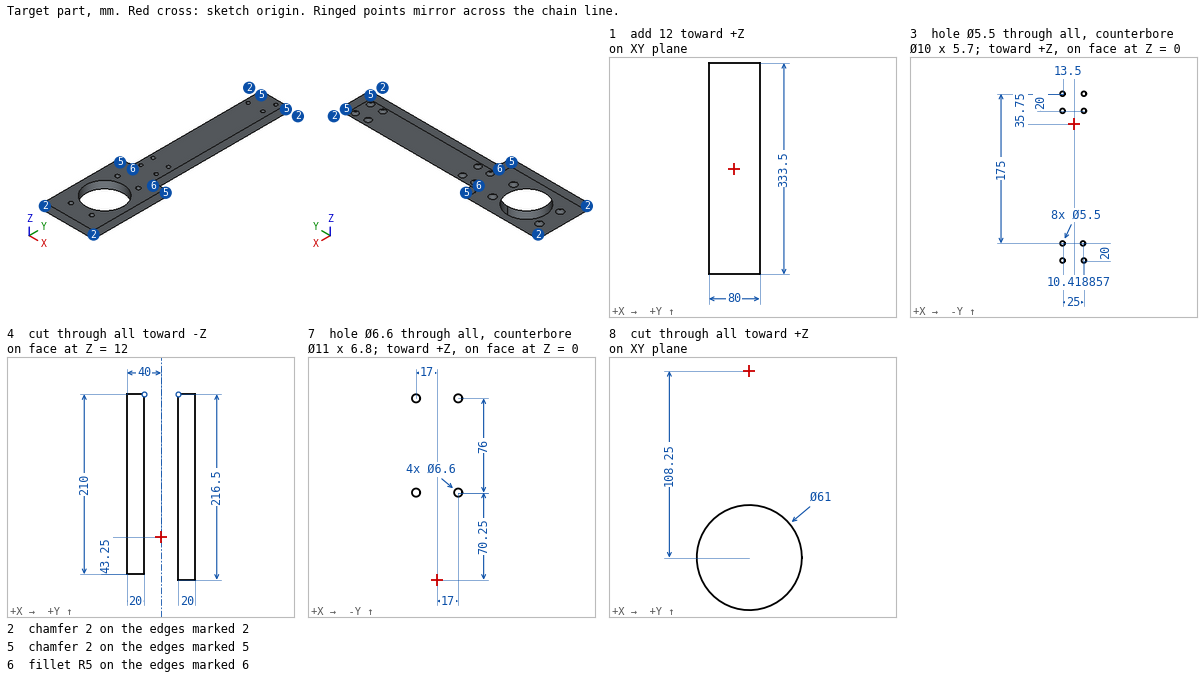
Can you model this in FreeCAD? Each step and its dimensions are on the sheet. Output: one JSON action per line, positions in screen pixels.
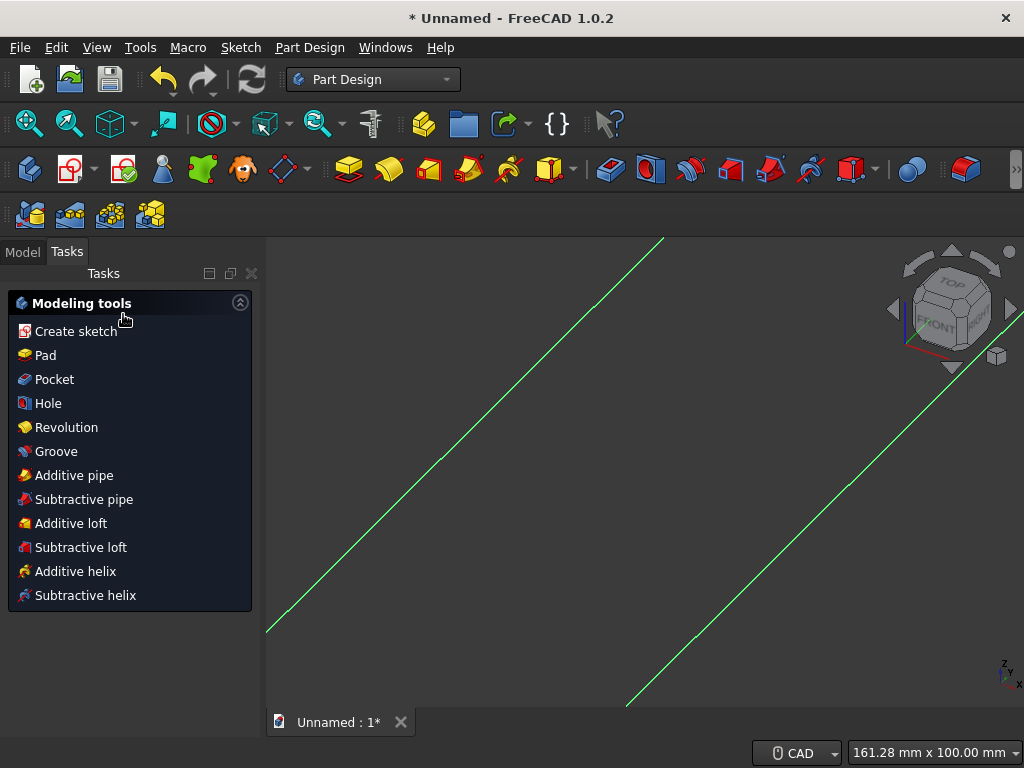
{"action": "left_click", "coordinate": [350, 170]}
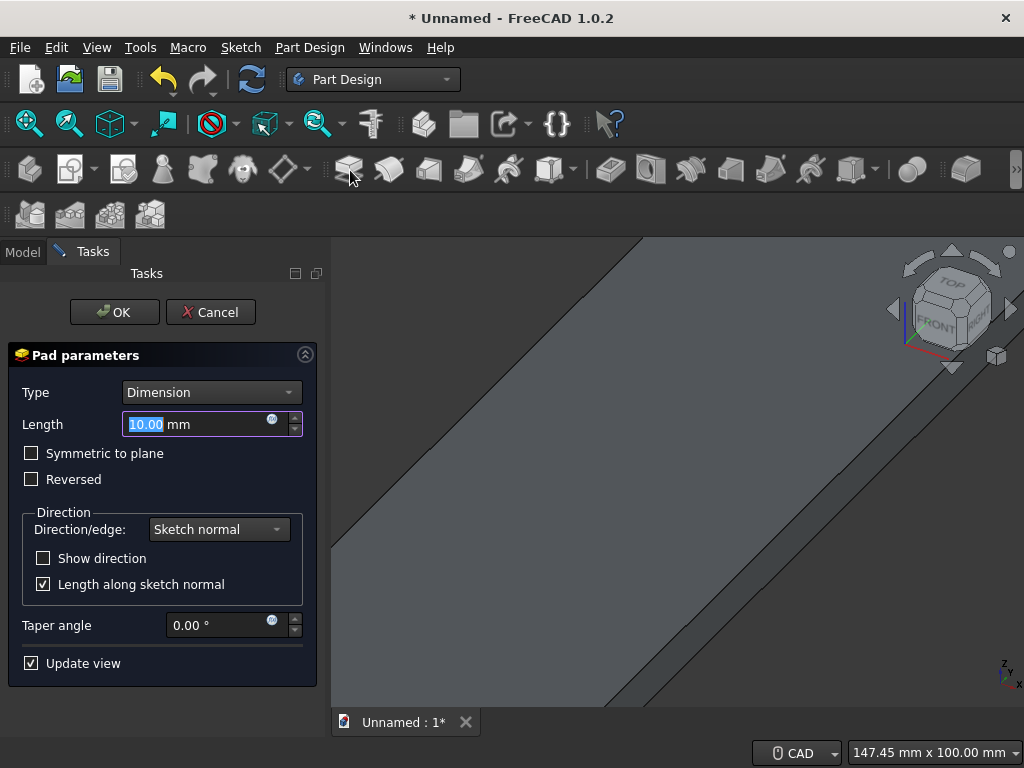
{"action": "type", "text": "12"}
{"action": "key", "text": "Tab"}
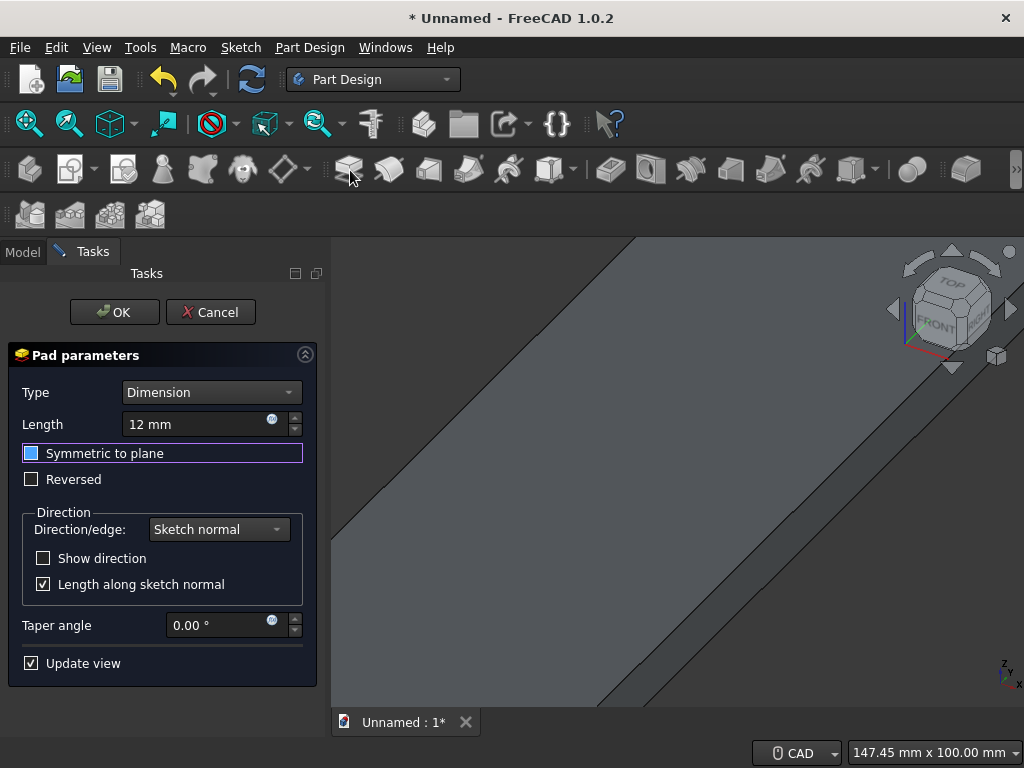
{"action": "left_click", "coordinate": [115, 312]}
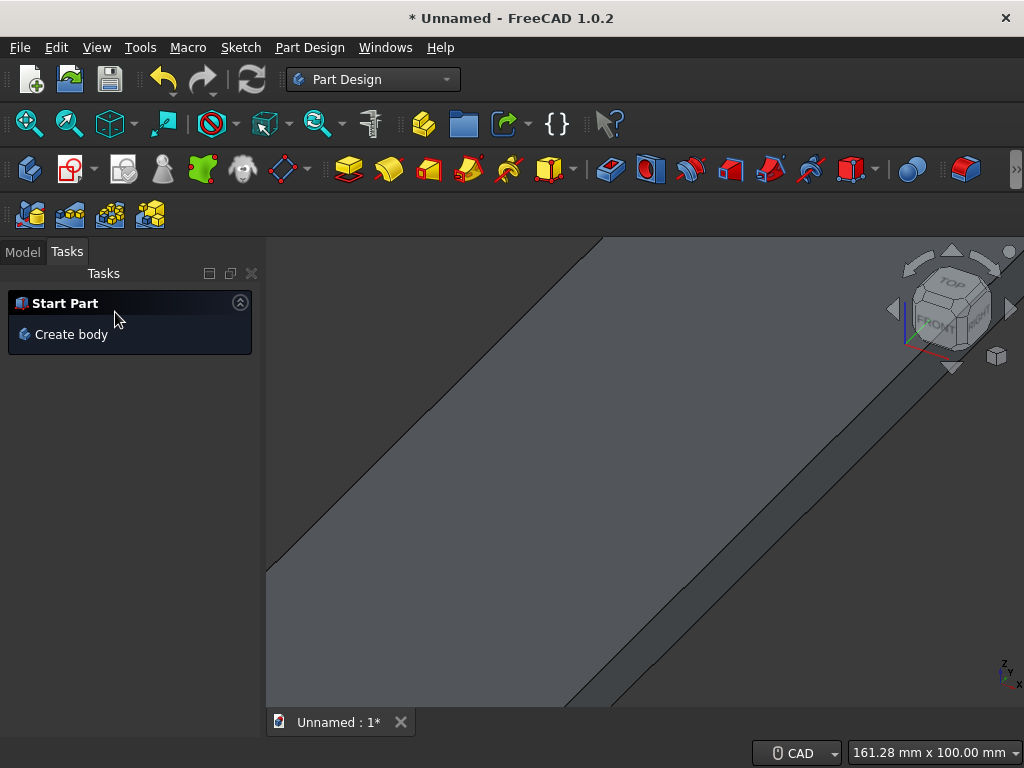
{"action": "left_click", "coordinate": [30, 124]}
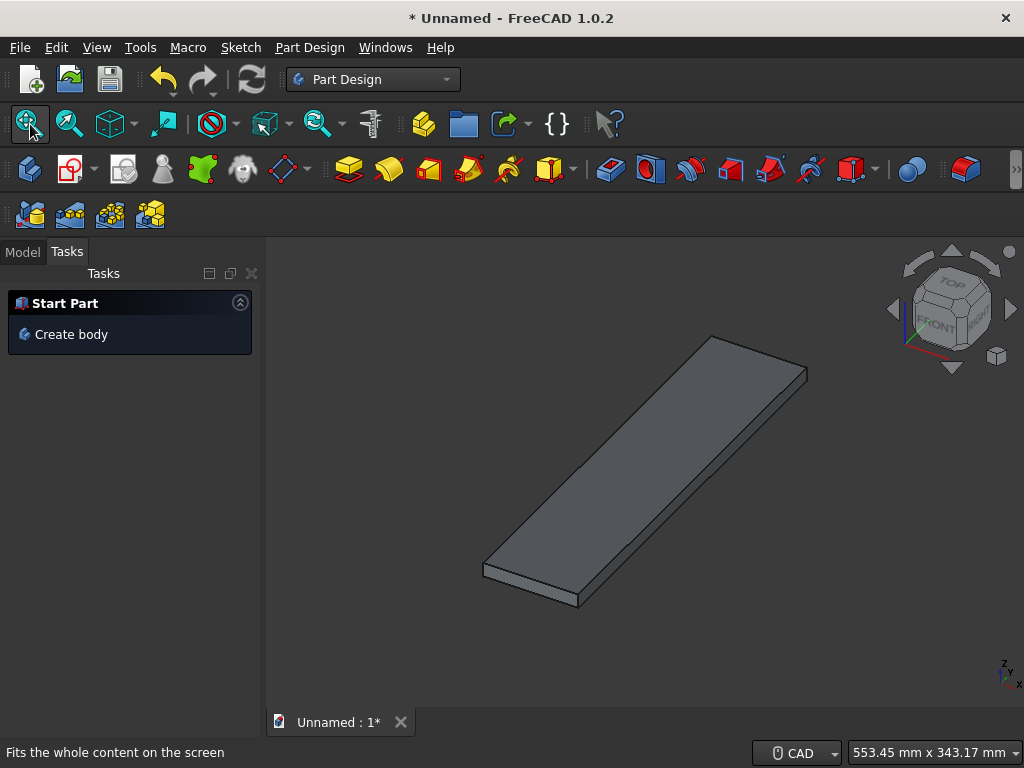
{"action": "left_click", "coordinate": [578, 600]}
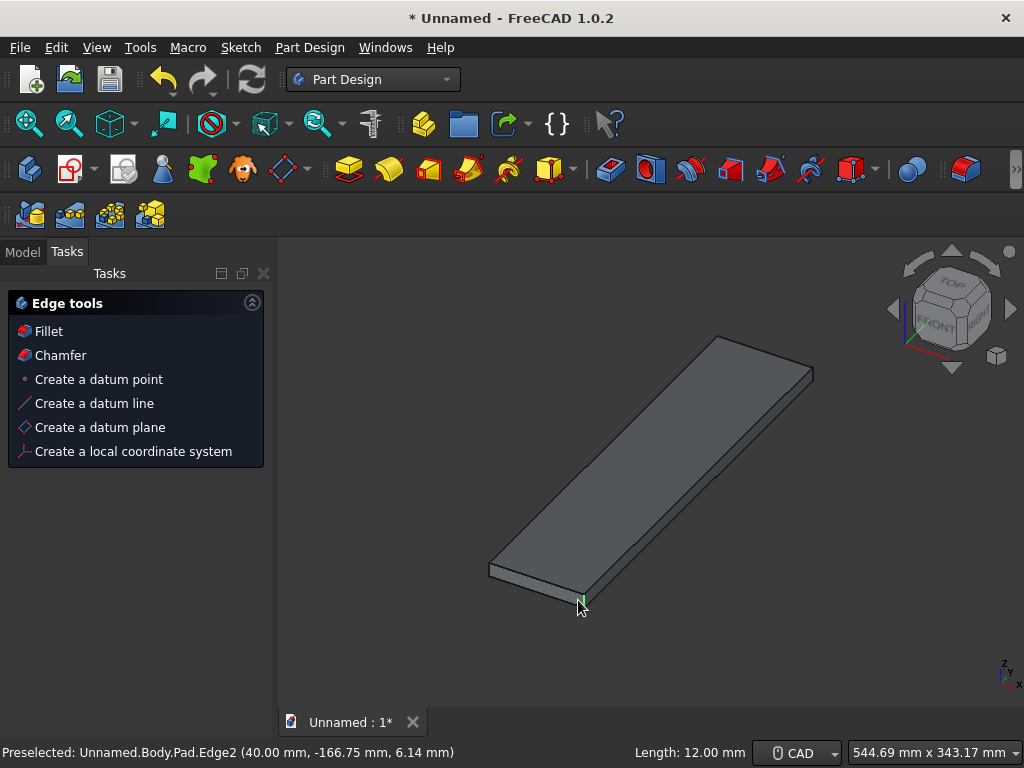
{"action": "scroll", "coordinate": [489, 569], "scroll_direction": "up", "scroll_amount": 5}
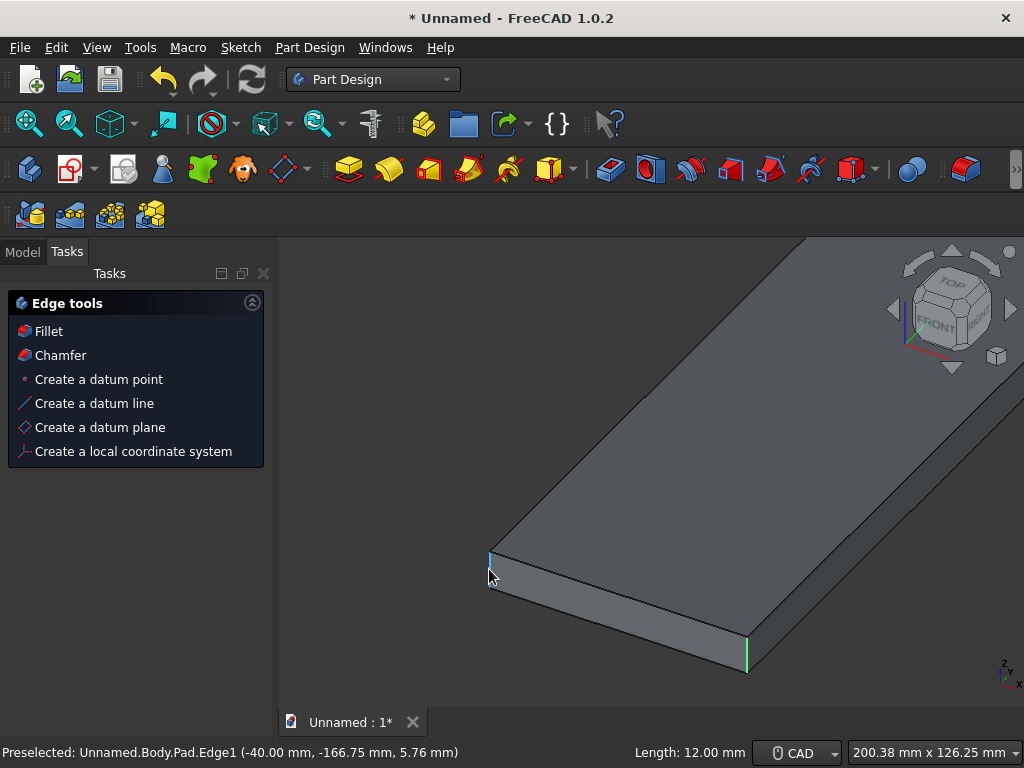
{"action": "key", "text": "v f"}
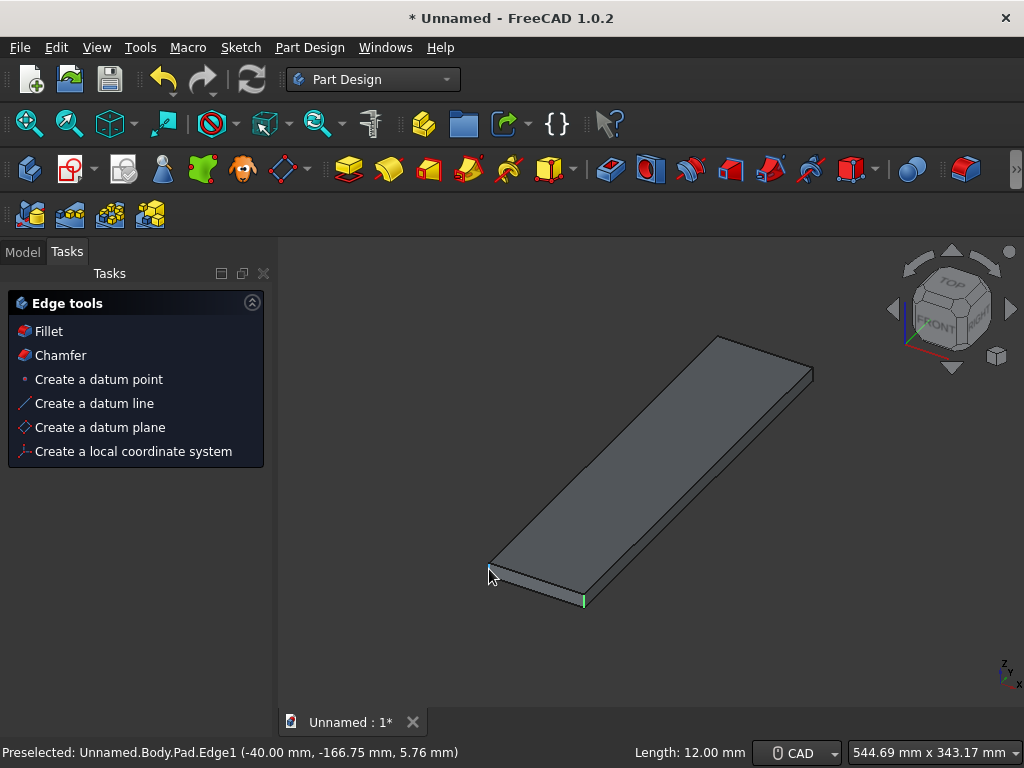
{"action": "key", "text": "0"}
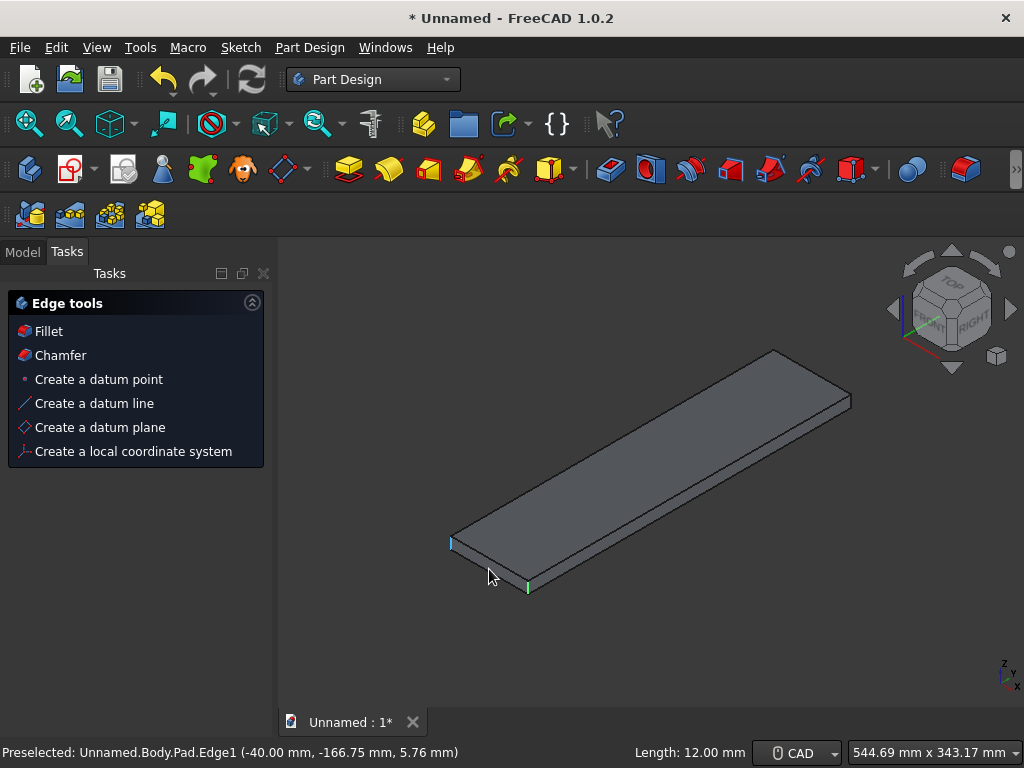
{"action": "scroll", "coordinate": [451, 542], "scroll_direction": "up", "scroll_amount": 5}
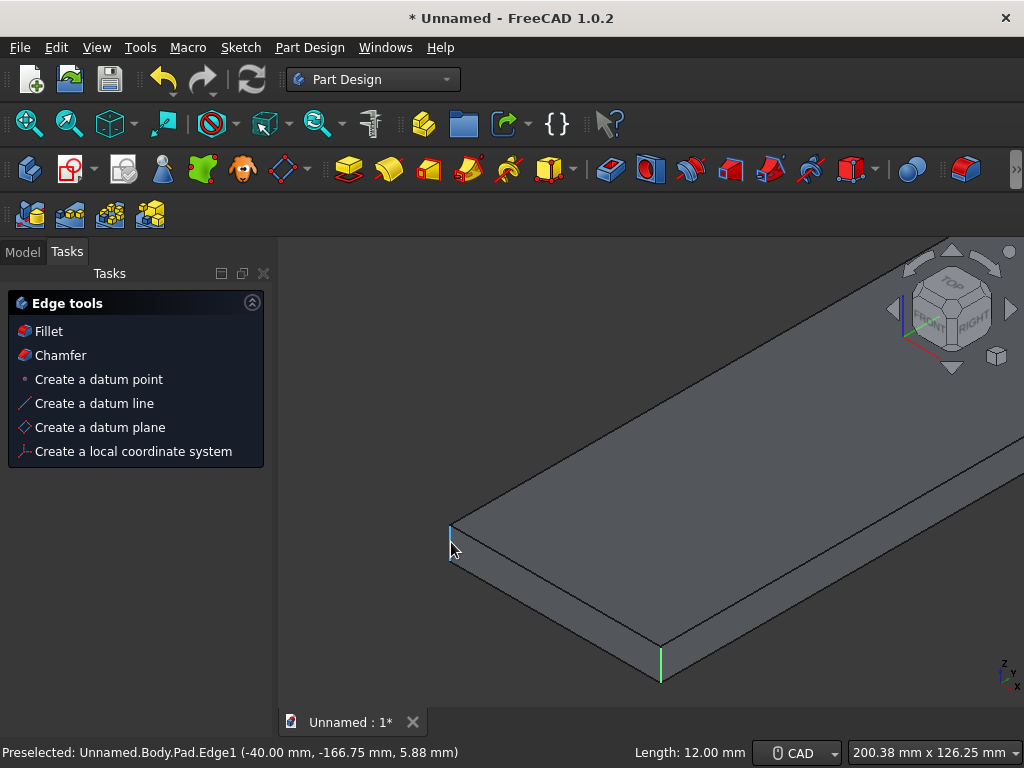
{"action": "key", "text": "v f"}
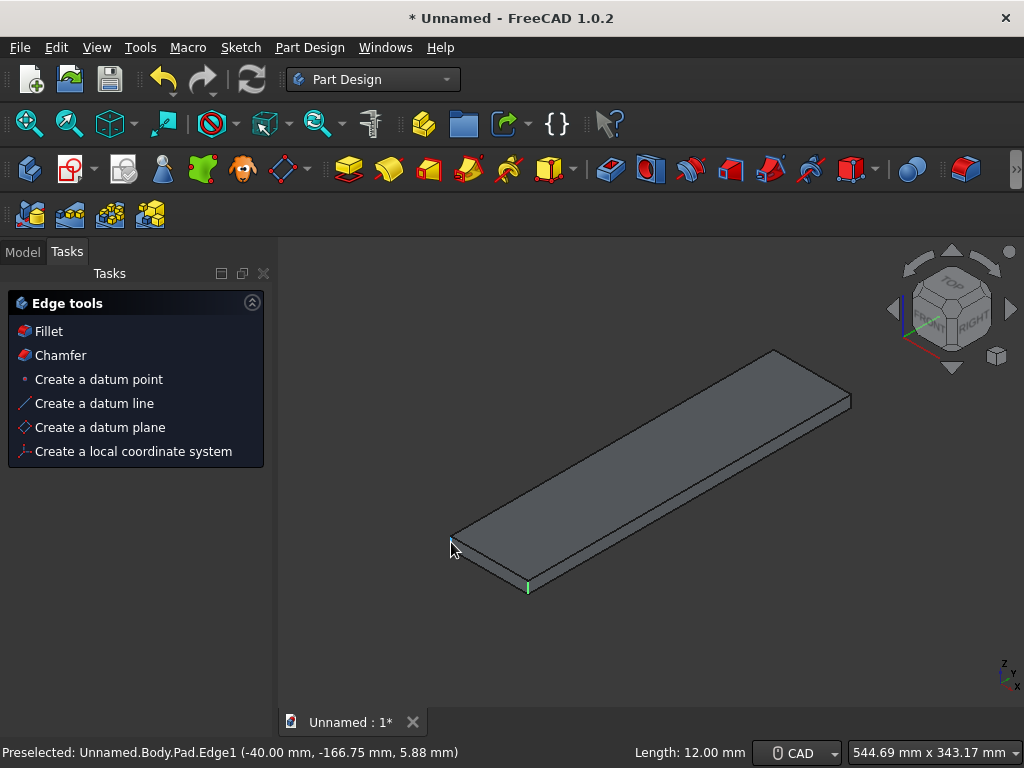
{"action": "key", "text": "2"}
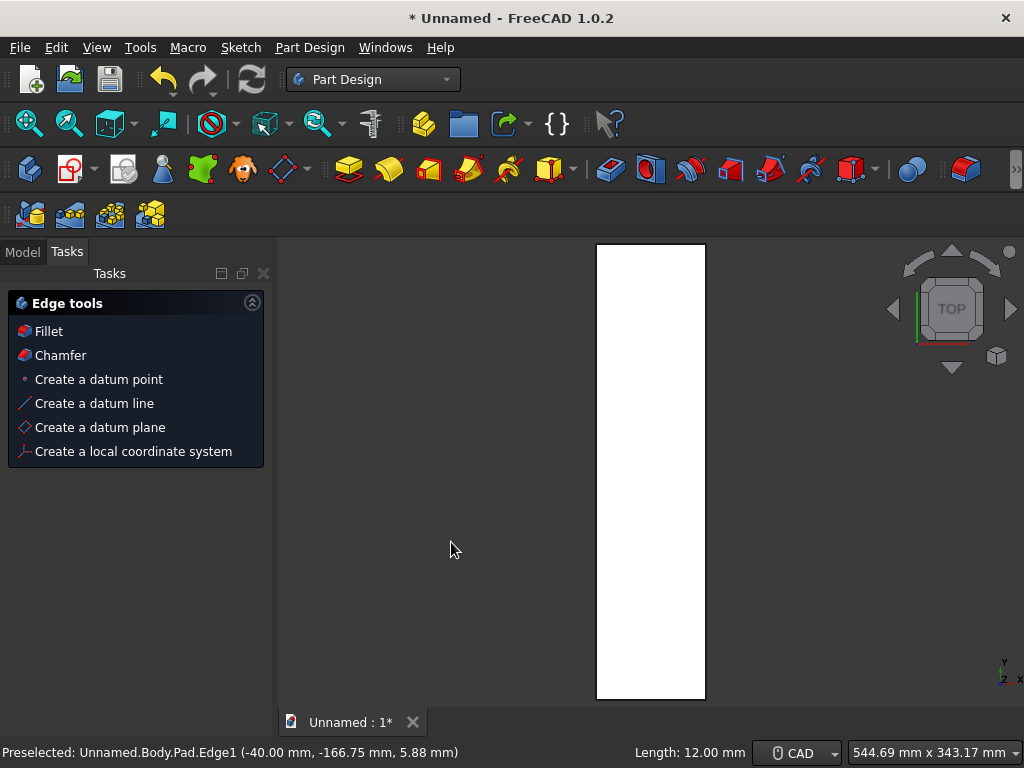
{"action": "key", "text": "1"}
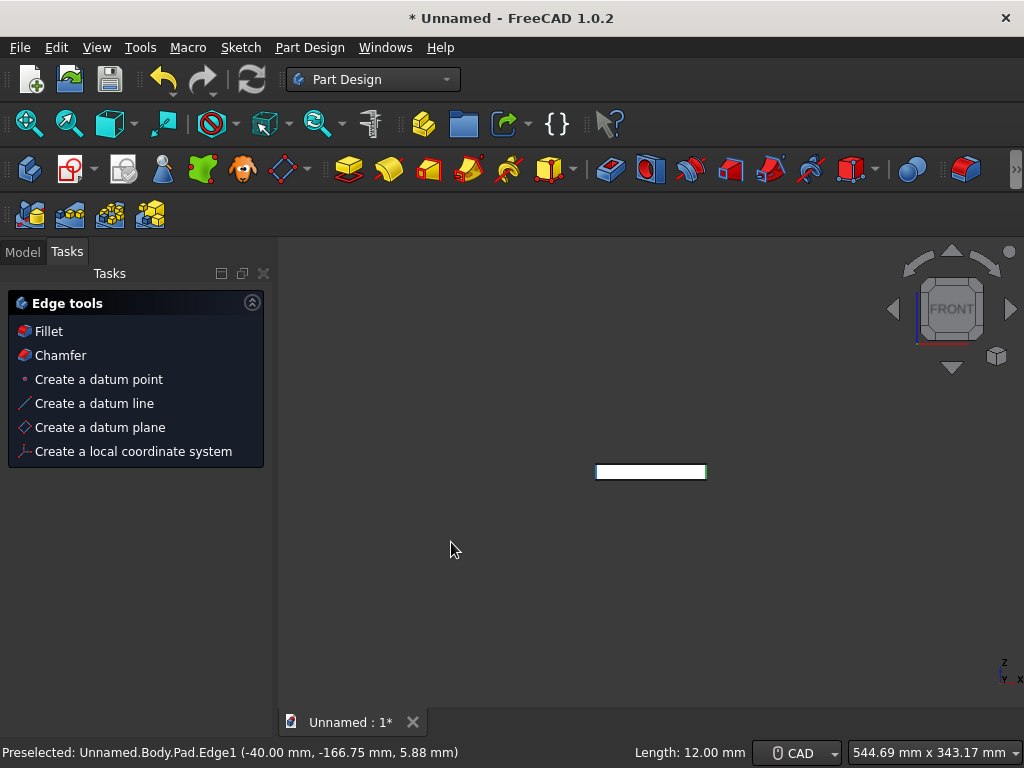
{"action": "key", "text": "v f"}